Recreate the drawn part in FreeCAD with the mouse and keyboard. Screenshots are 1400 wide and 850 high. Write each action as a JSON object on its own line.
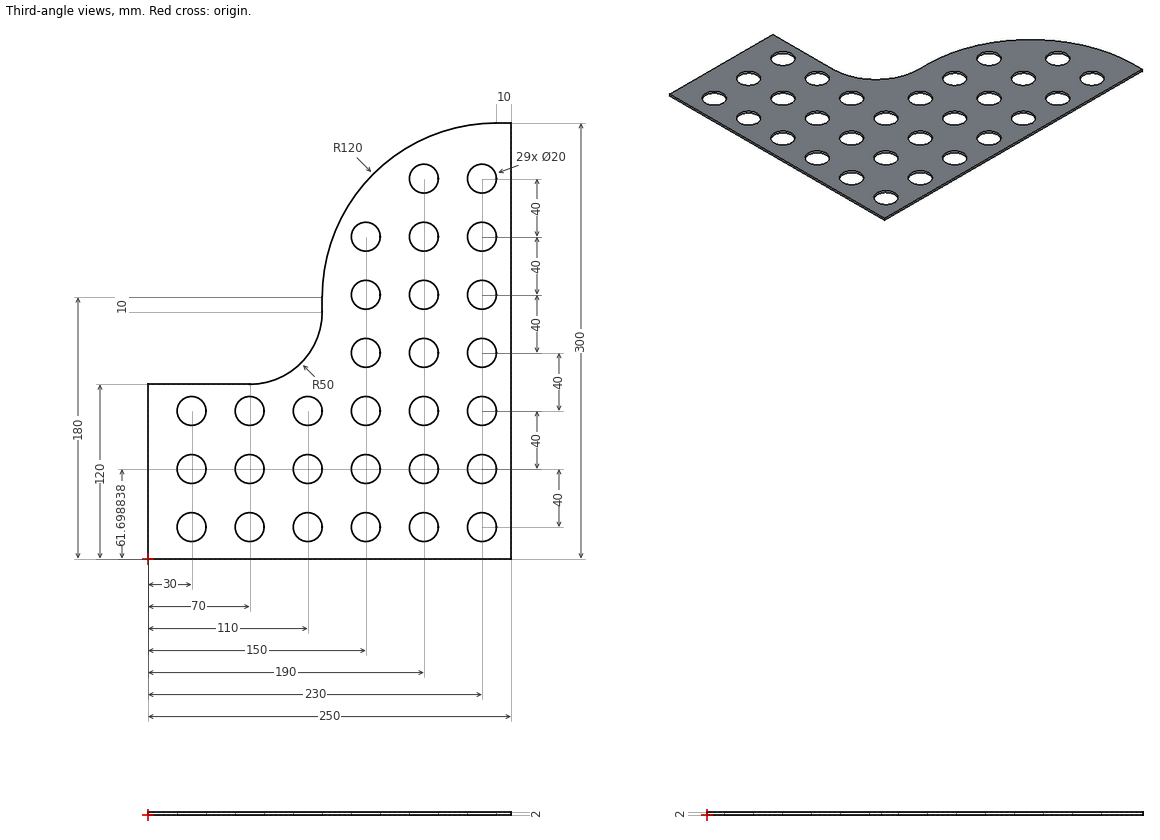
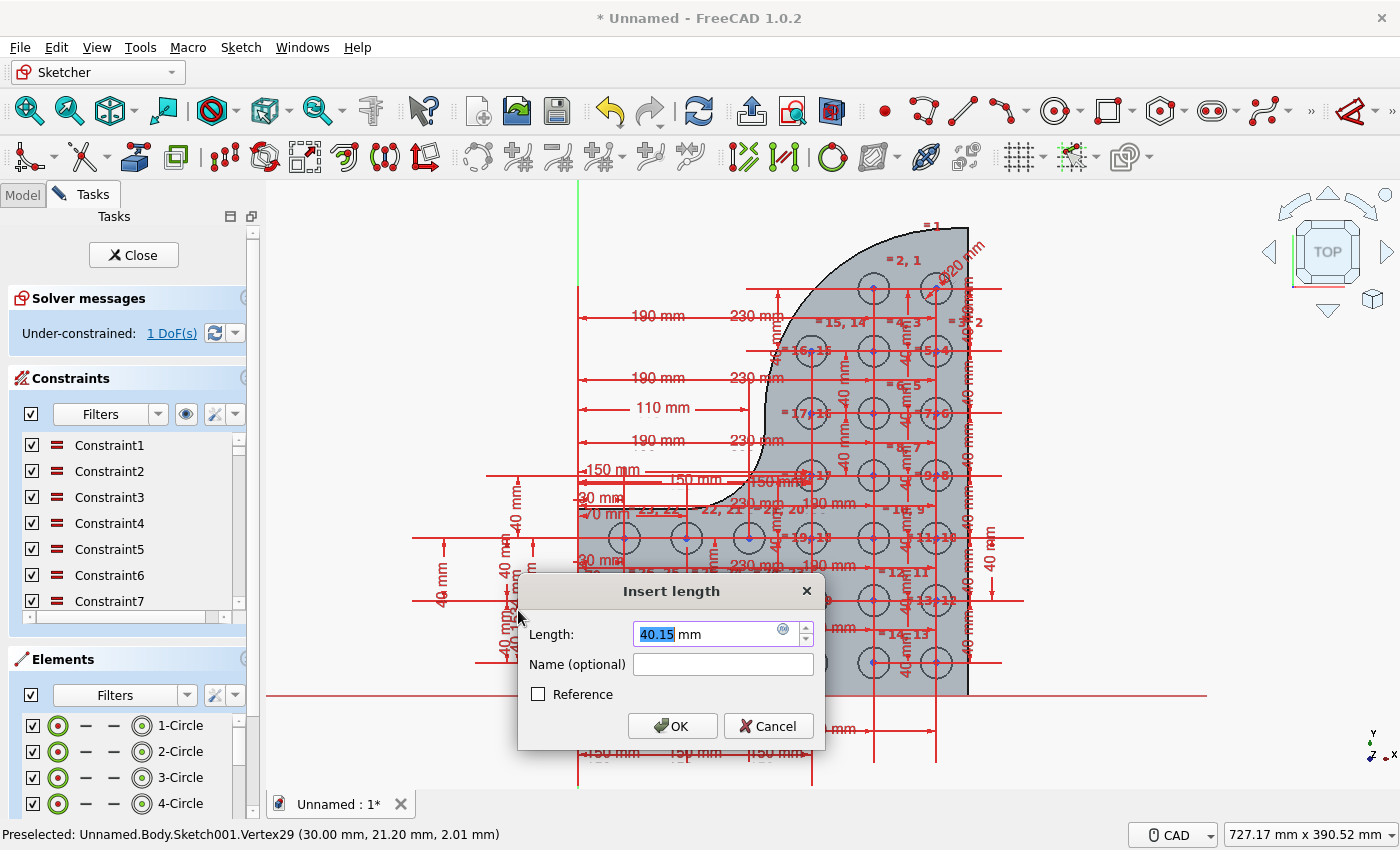
{"action": "type", "text": "40"}
{"action": "key", "text": "Return"}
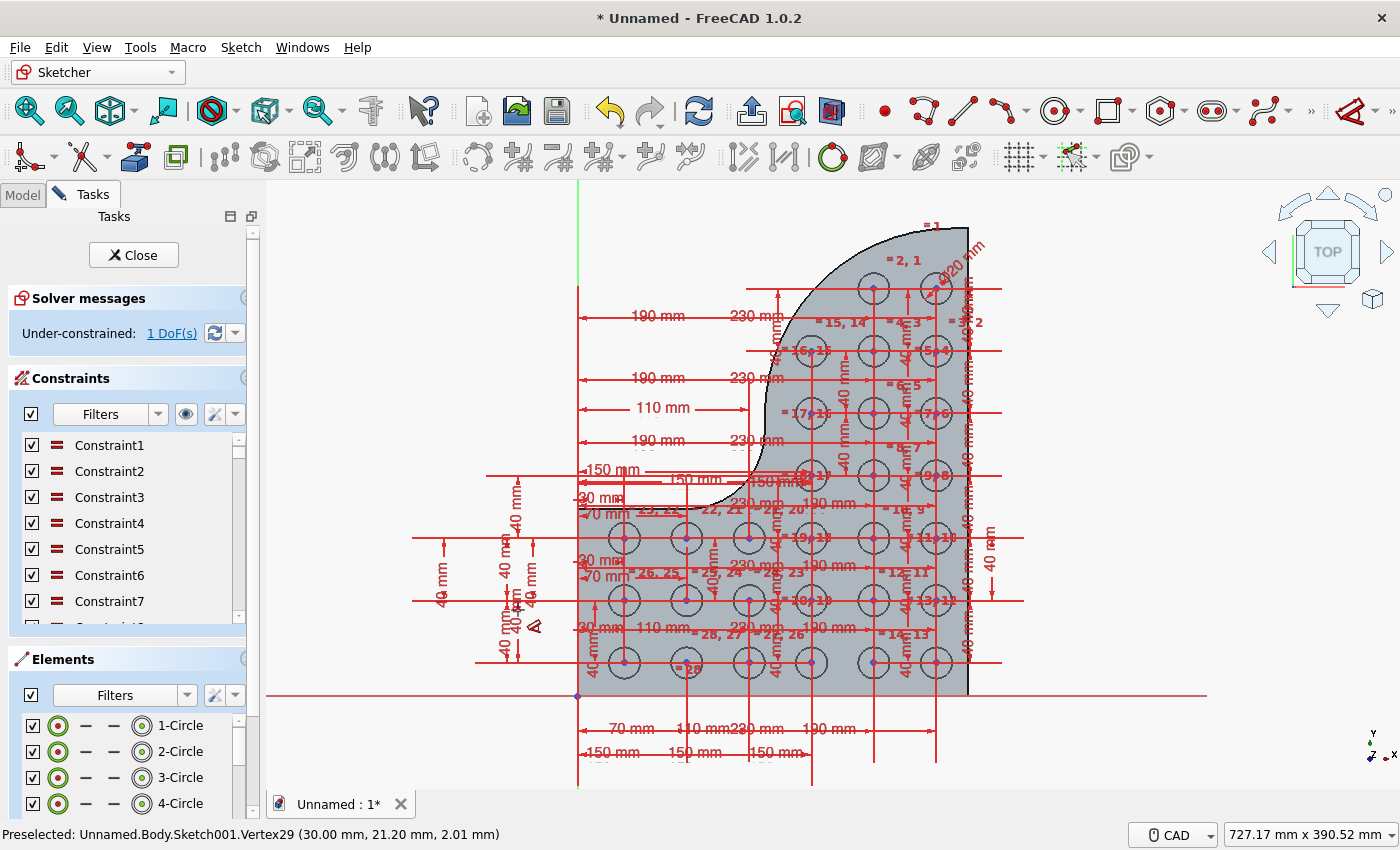
{"action": "left_click", "coordinate": [936, 601]}
{"action": "left_click", "coordinate": [544, 682]}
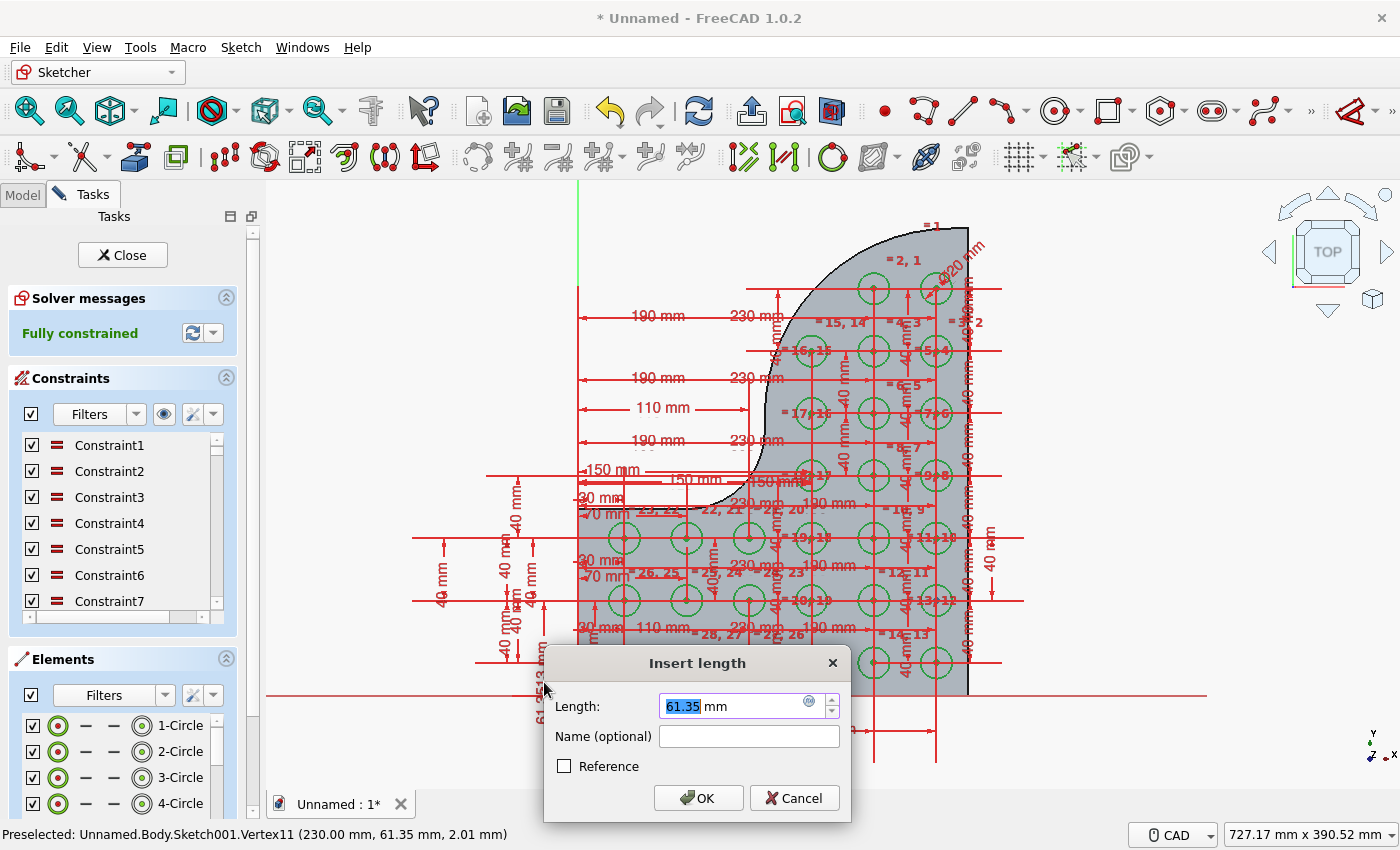
{"action": "type", "text": "61.698838"}
{"action": "key", "text": "Return"}
{"action": "key", "text": "Escape"}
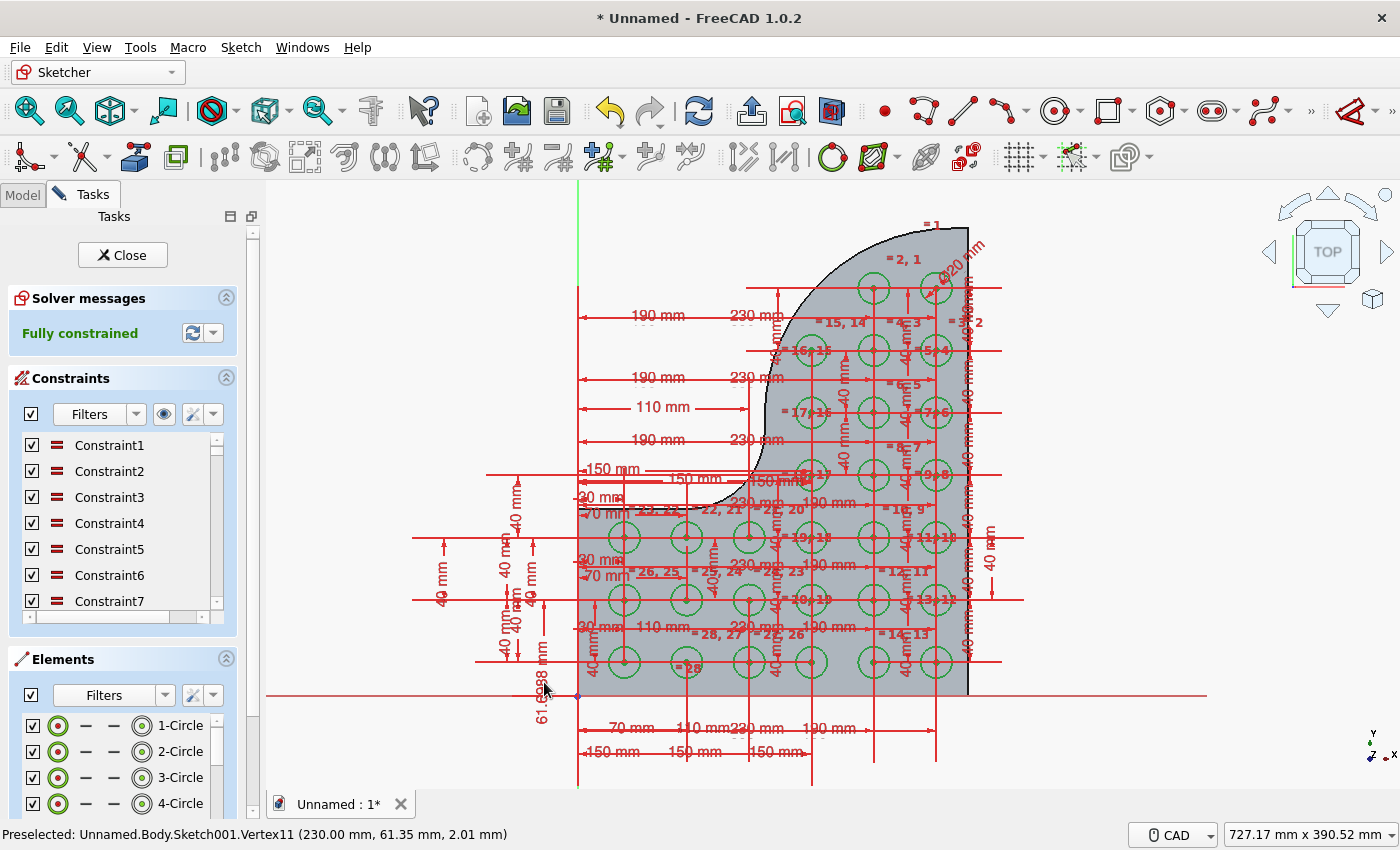
{"action": "left_click", "coordinate": [123, 255]}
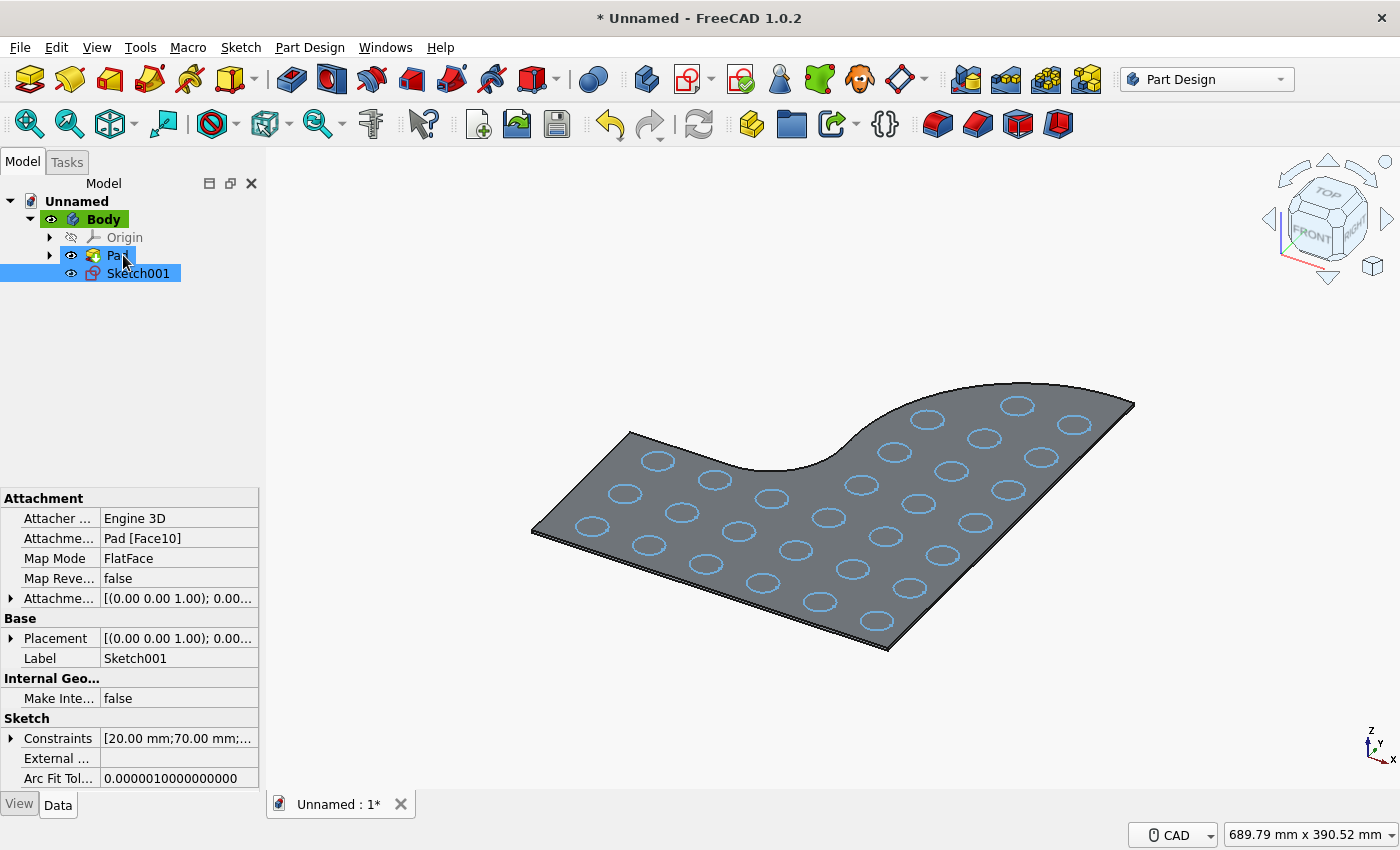
{"action": "left_click", "coordinate": [292, 80]}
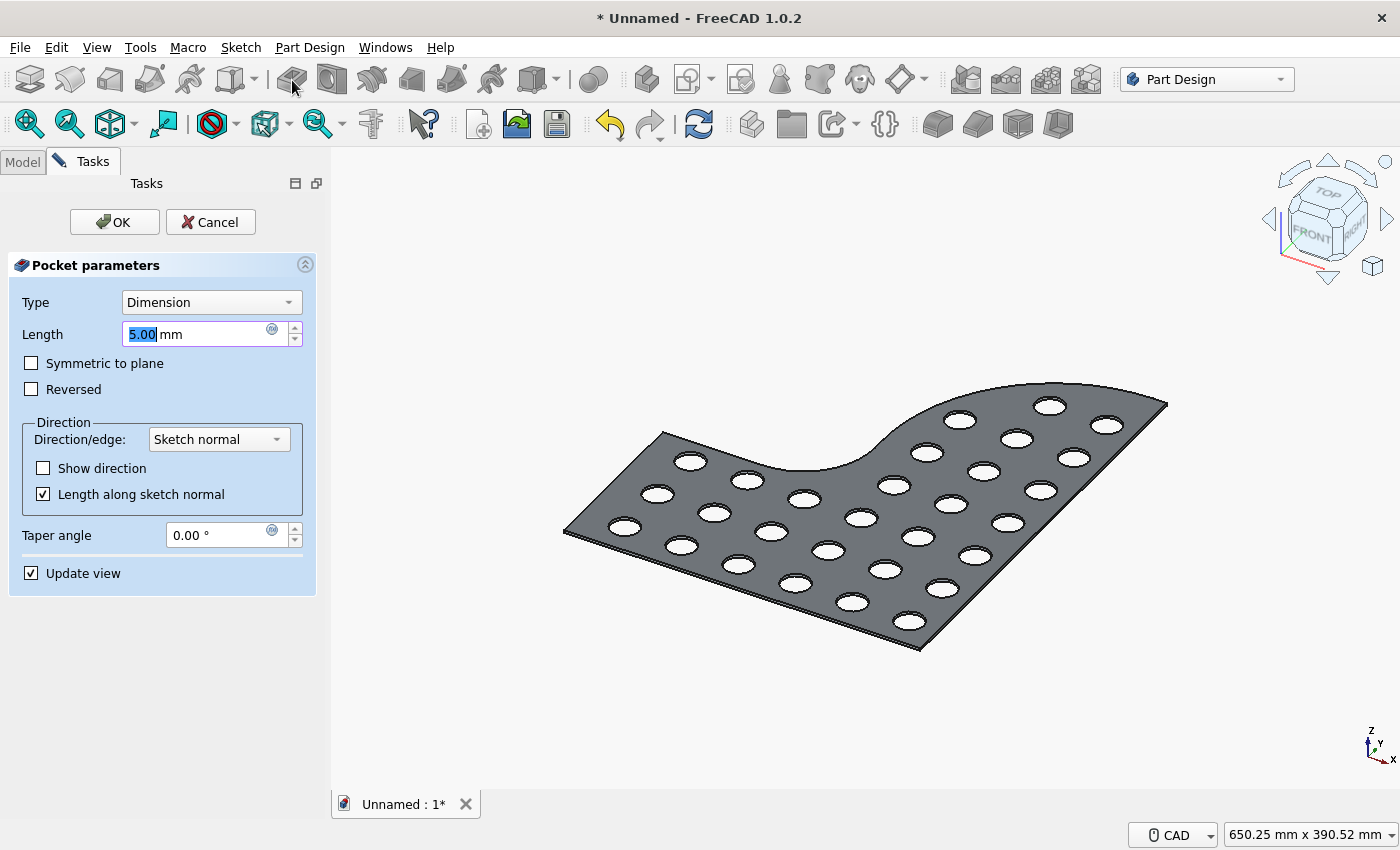
{"action": "type", "text": "2"}
{"action": "key", "text": "Tab"}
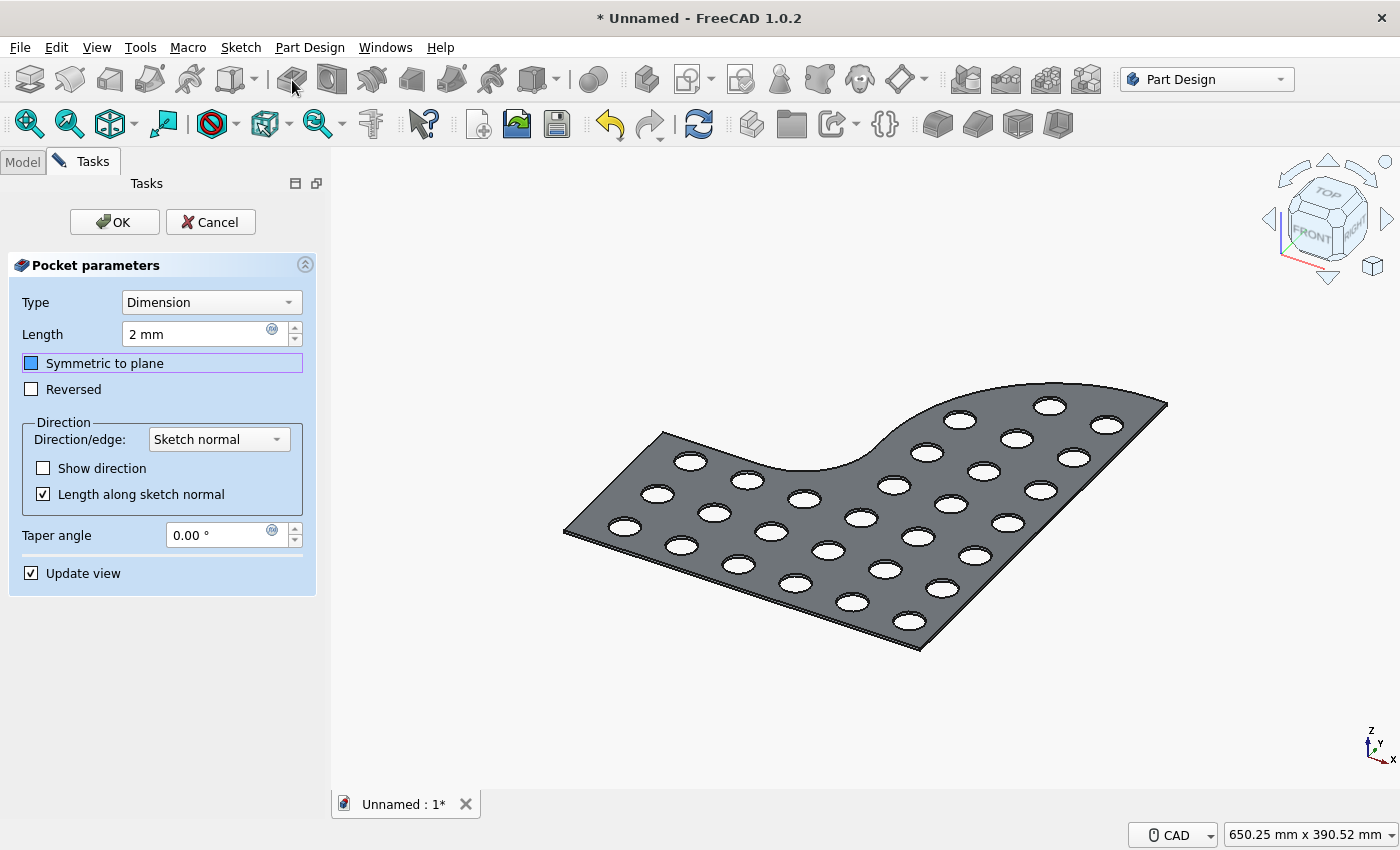
{"action": "left_click", "coordinate": [115, 222]}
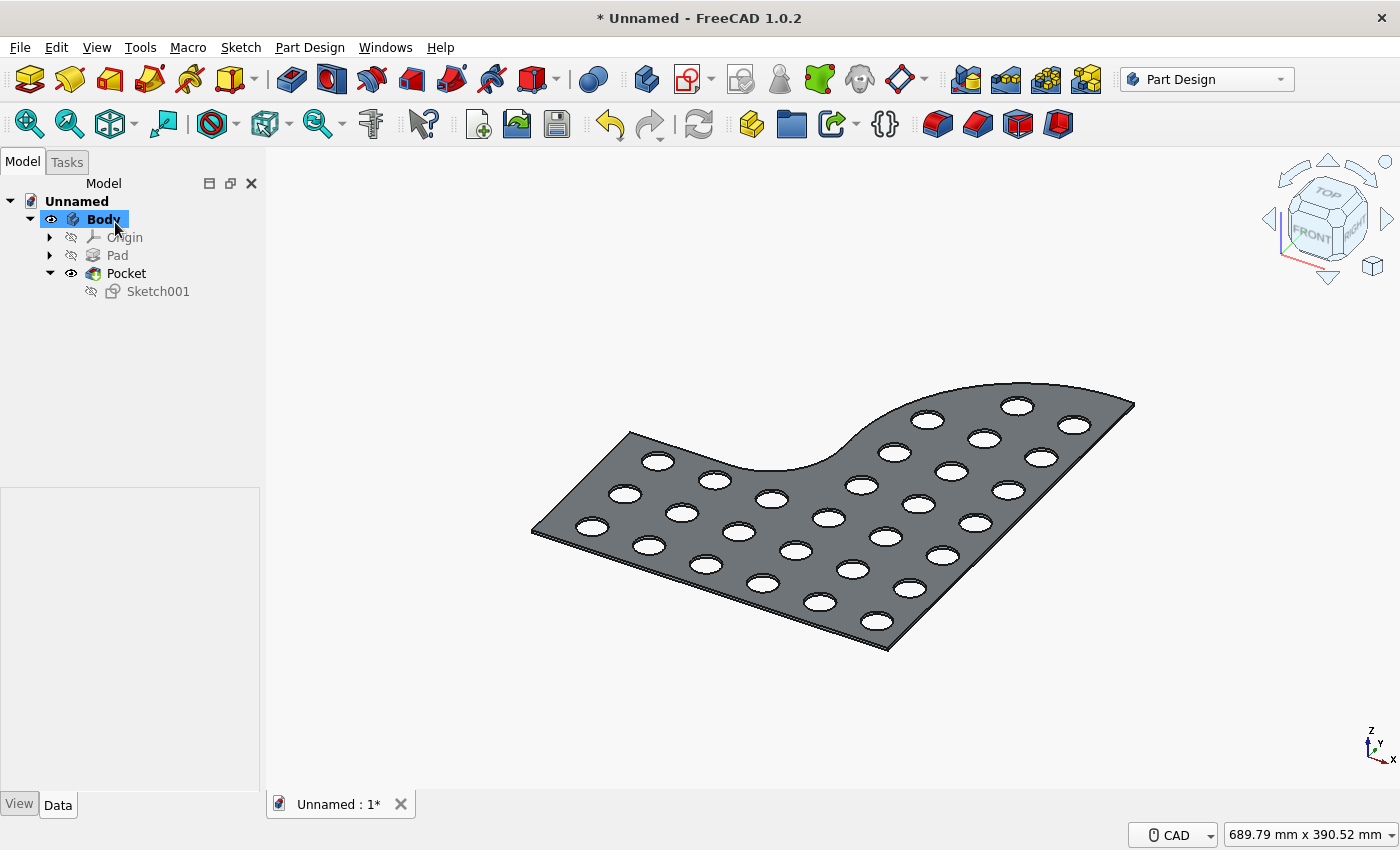
{"action": "key", "text": "0"}